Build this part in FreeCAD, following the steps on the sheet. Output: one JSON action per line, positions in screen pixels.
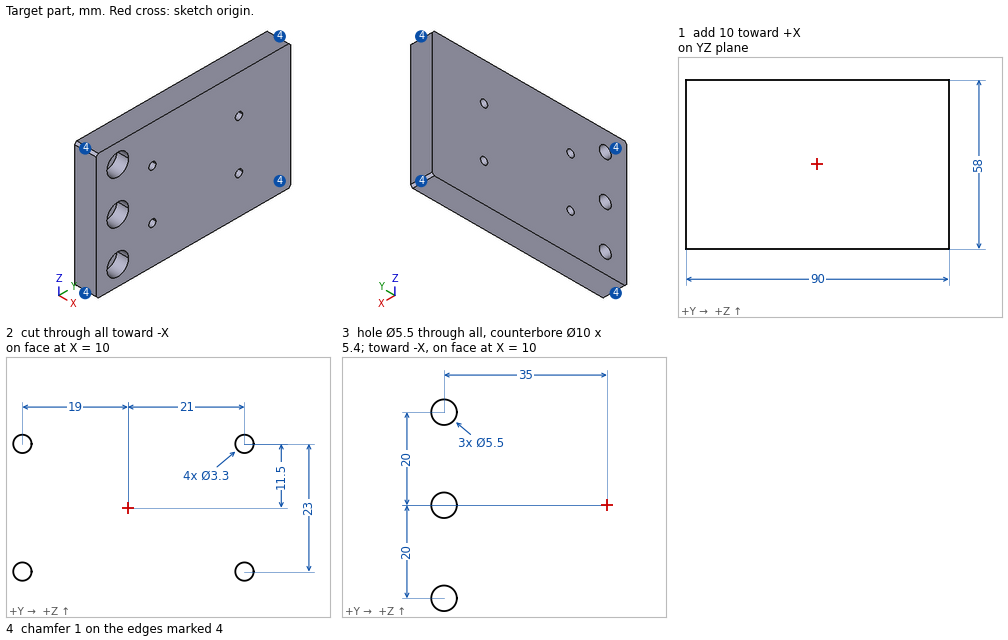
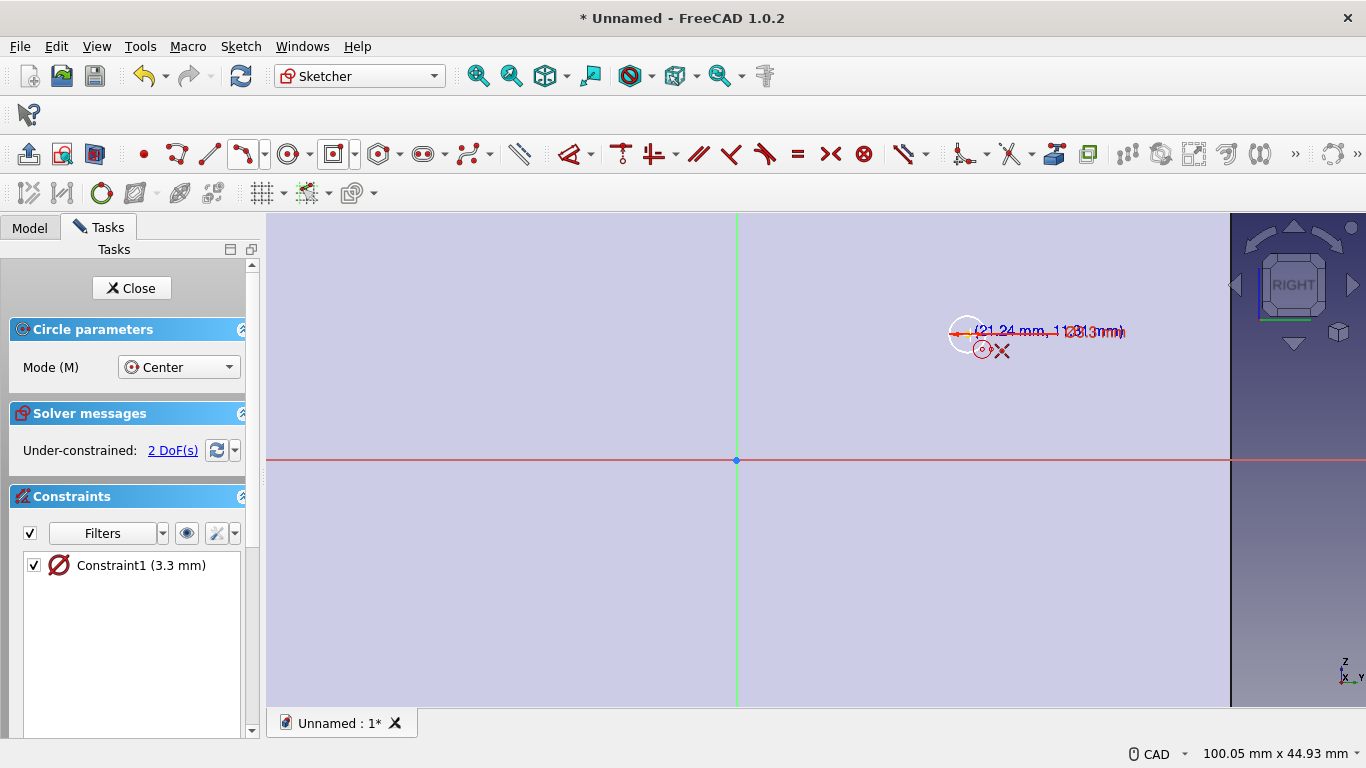
{"action": "scroll", "coordinate": [968, 586], "scroll_direction": "up", "scroll_amount": 2}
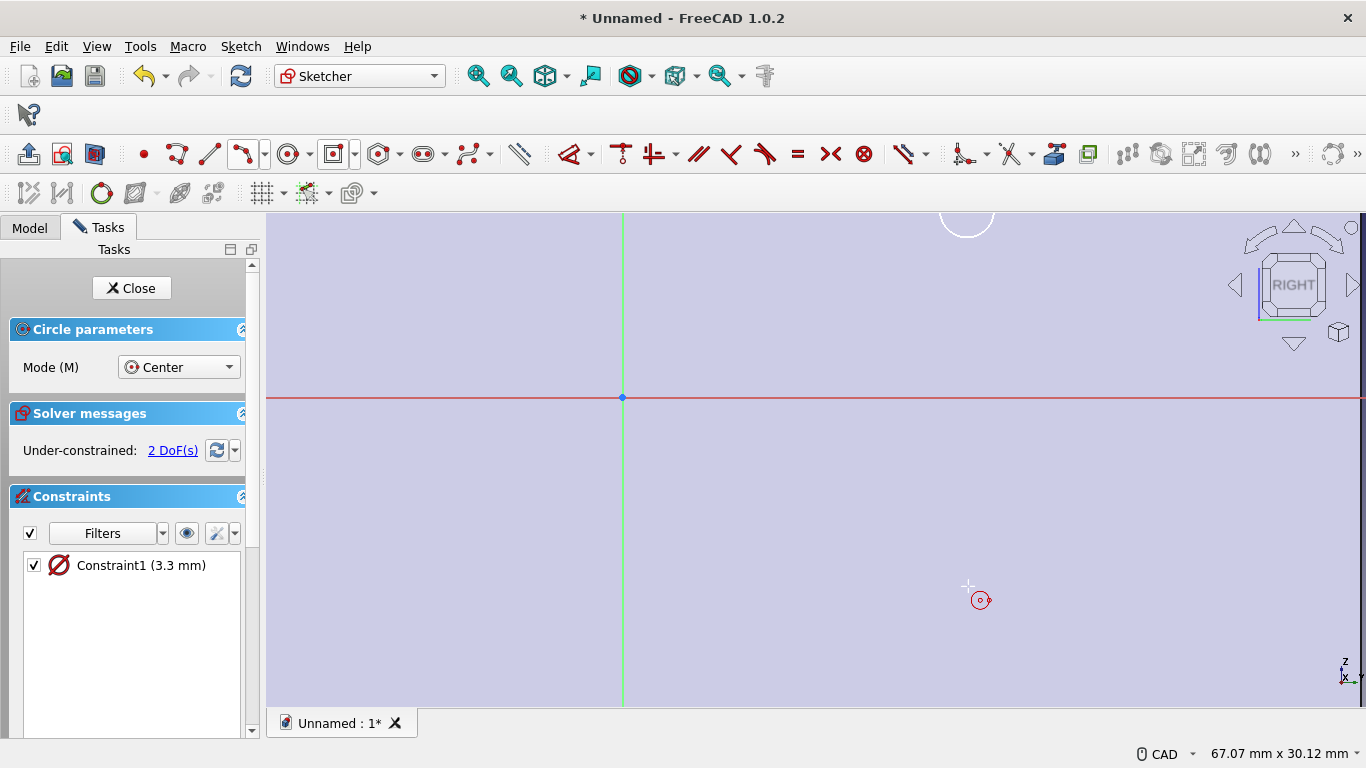
{"action": "left_click", "coordinate": [967, 586]}
{"action": "mouse_move", "coordinate": [986, 567]}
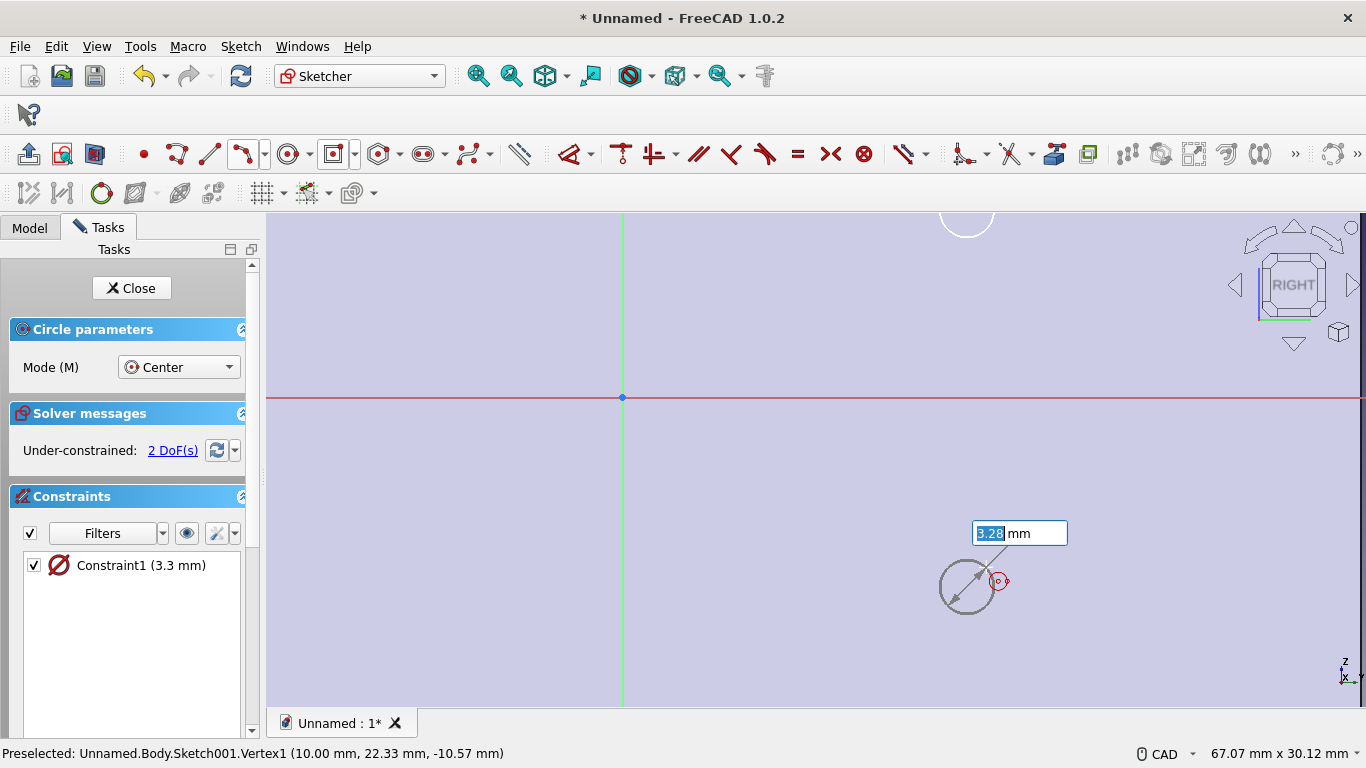
{"action": "type", "text": "3.3"}
{"action": "key", "text": "Return"}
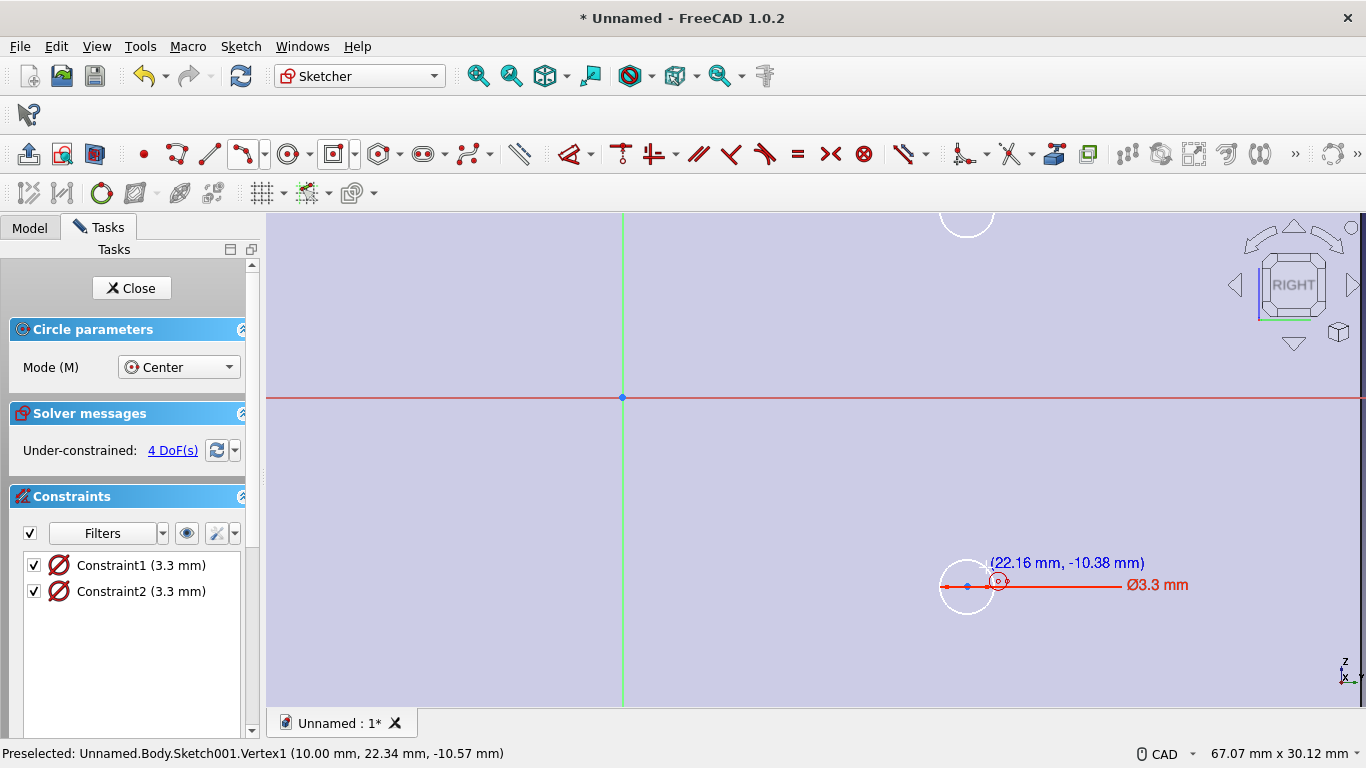
{"action": "scroll", "coordinate": [968, 587], "scroll_direction": "down", "scroll_amount": 2}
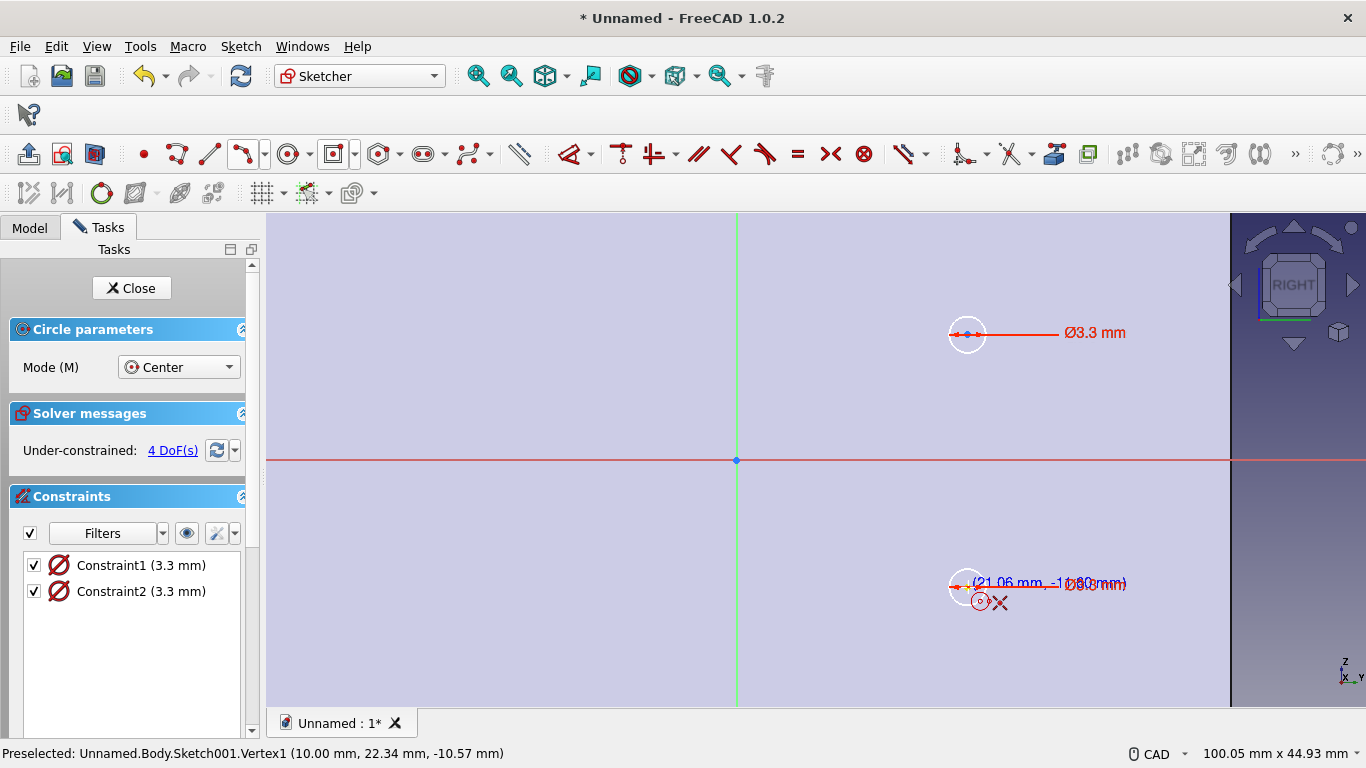
{"action": "scroll", "coordinate": [528, 334], "scroll_direction": "up", "scroll_amount": 2}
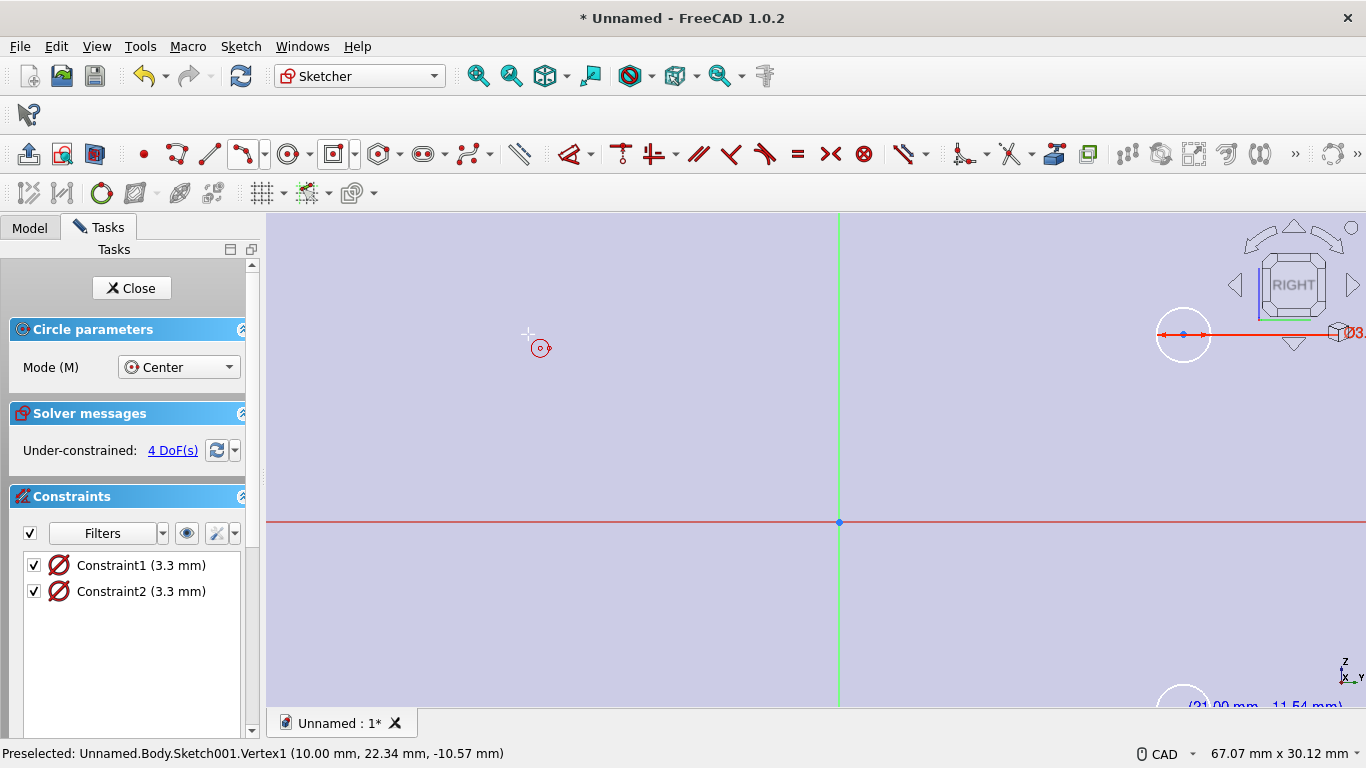
{"action": "left_click", "coordinate": [528, 334]}
{"action": "mouse_move", "coordinate": [547, 315]}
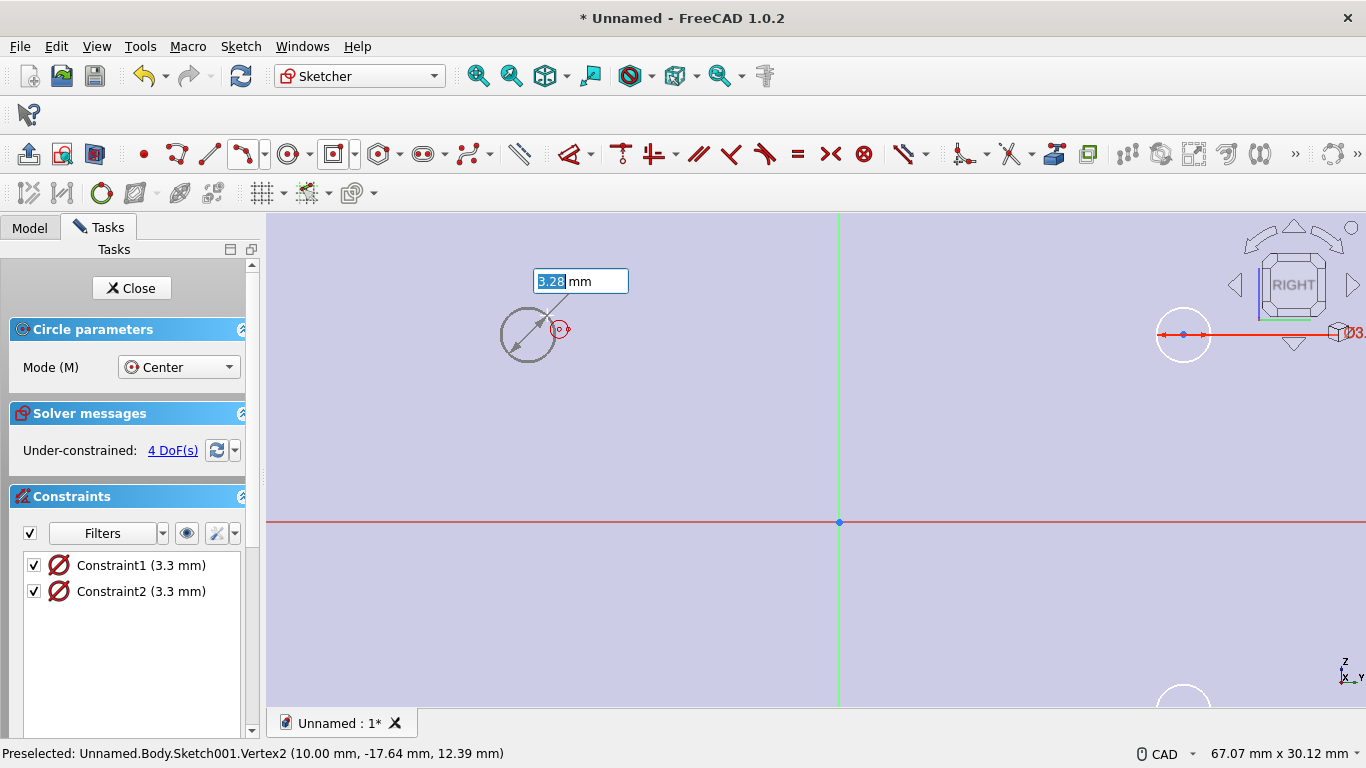
{"action": "type", "text": "3.3"}
{"action": "key", "text": "Return"}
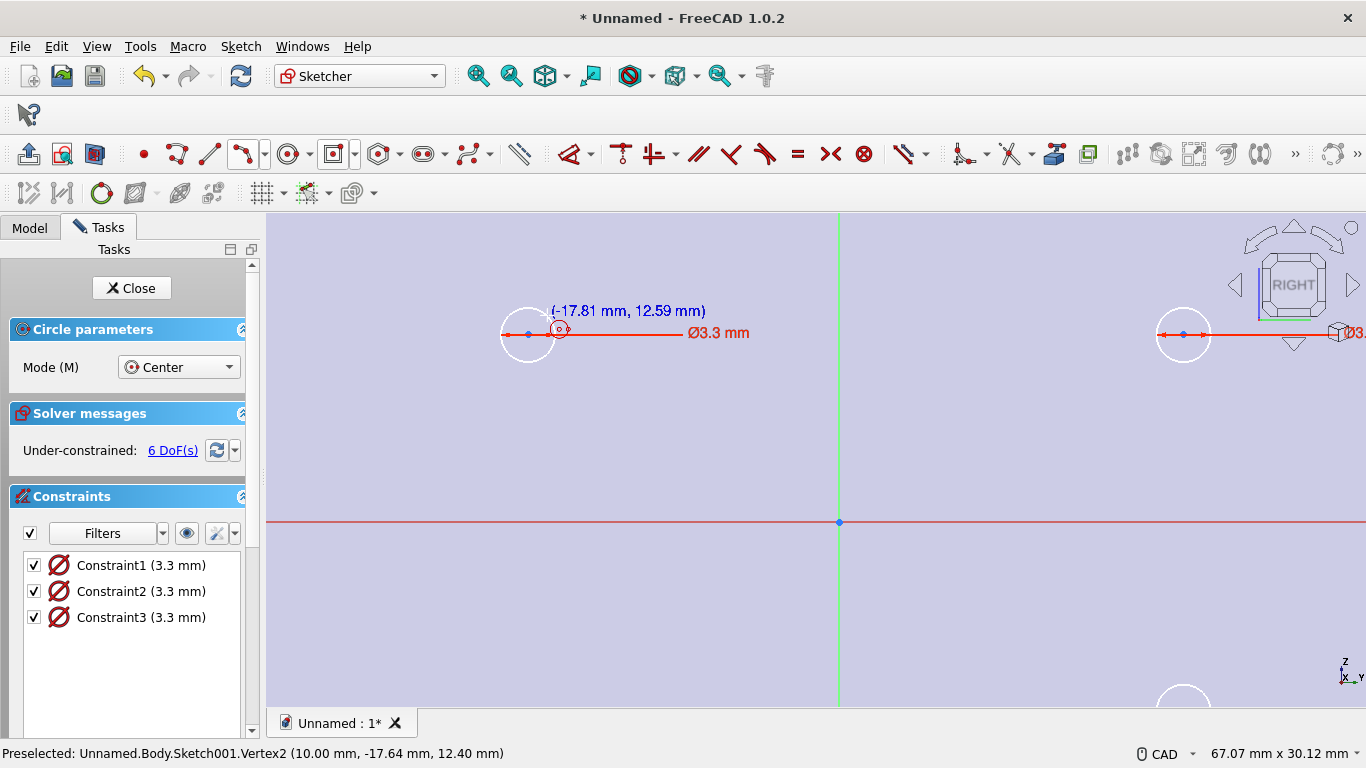
{"action": "scroll", "coordinate": [528, 333], "scroll_direction": "down", "scroll_amount": 2}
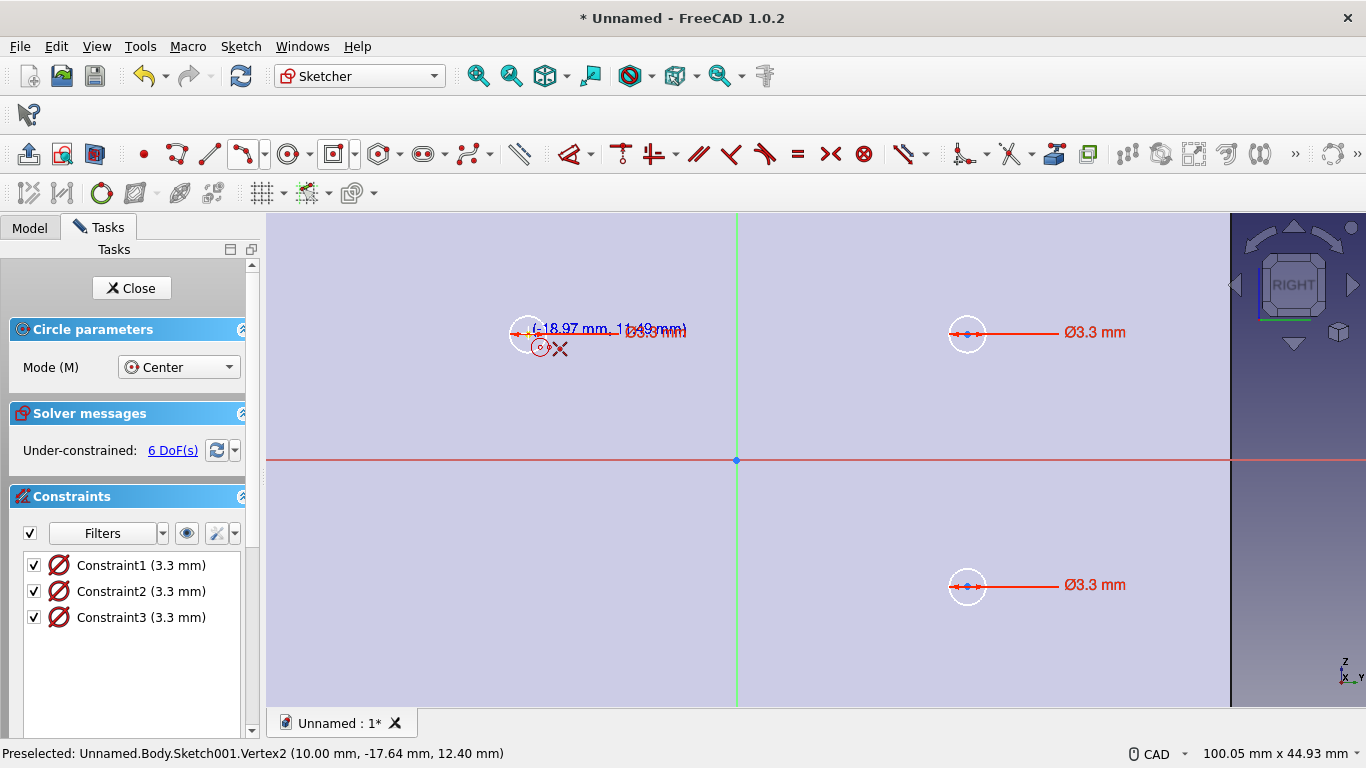
{"action": "scroll", "coordinate": [528, 586], "scroll_direction": "up", "scroll_amount": 2}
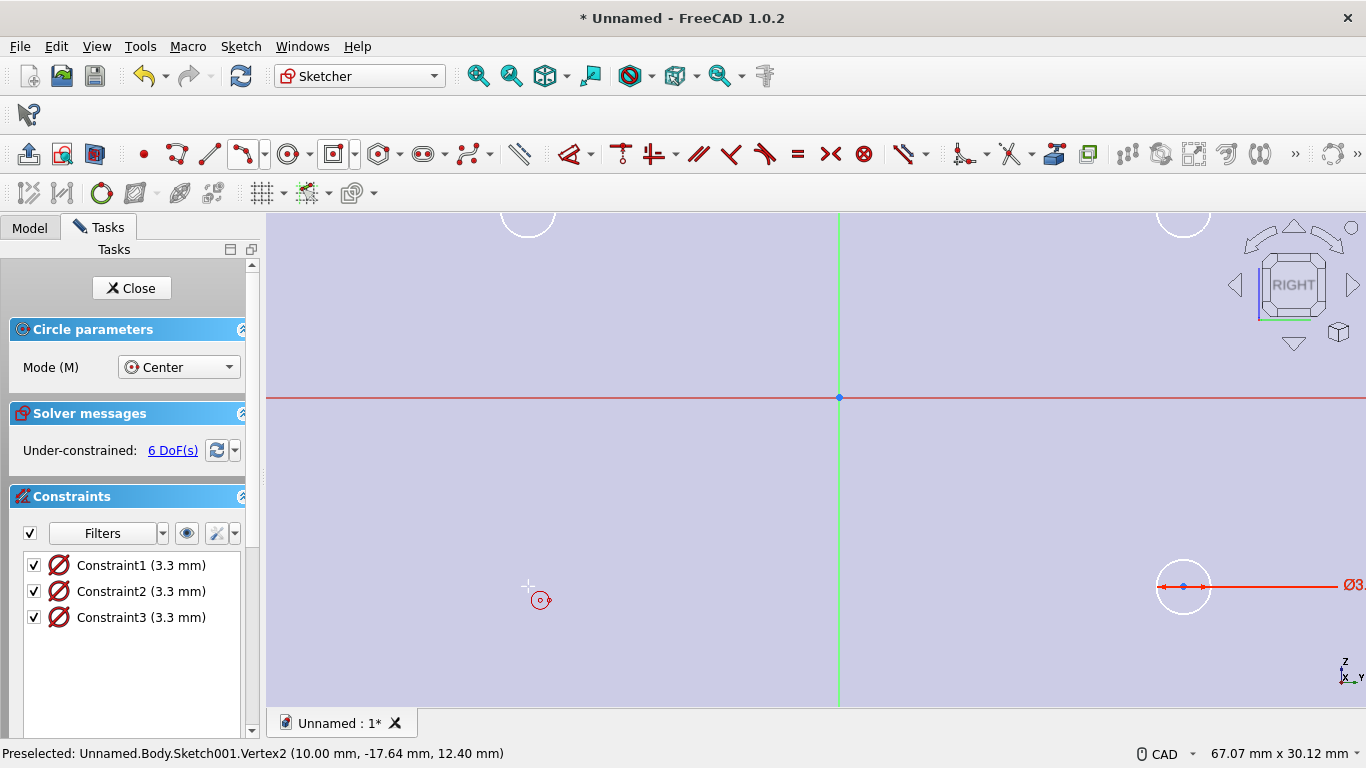
{"action": "left_click", "coordinate": [528, 586]}
{"action": "mouse_move", "coordinate": [547, 567]}